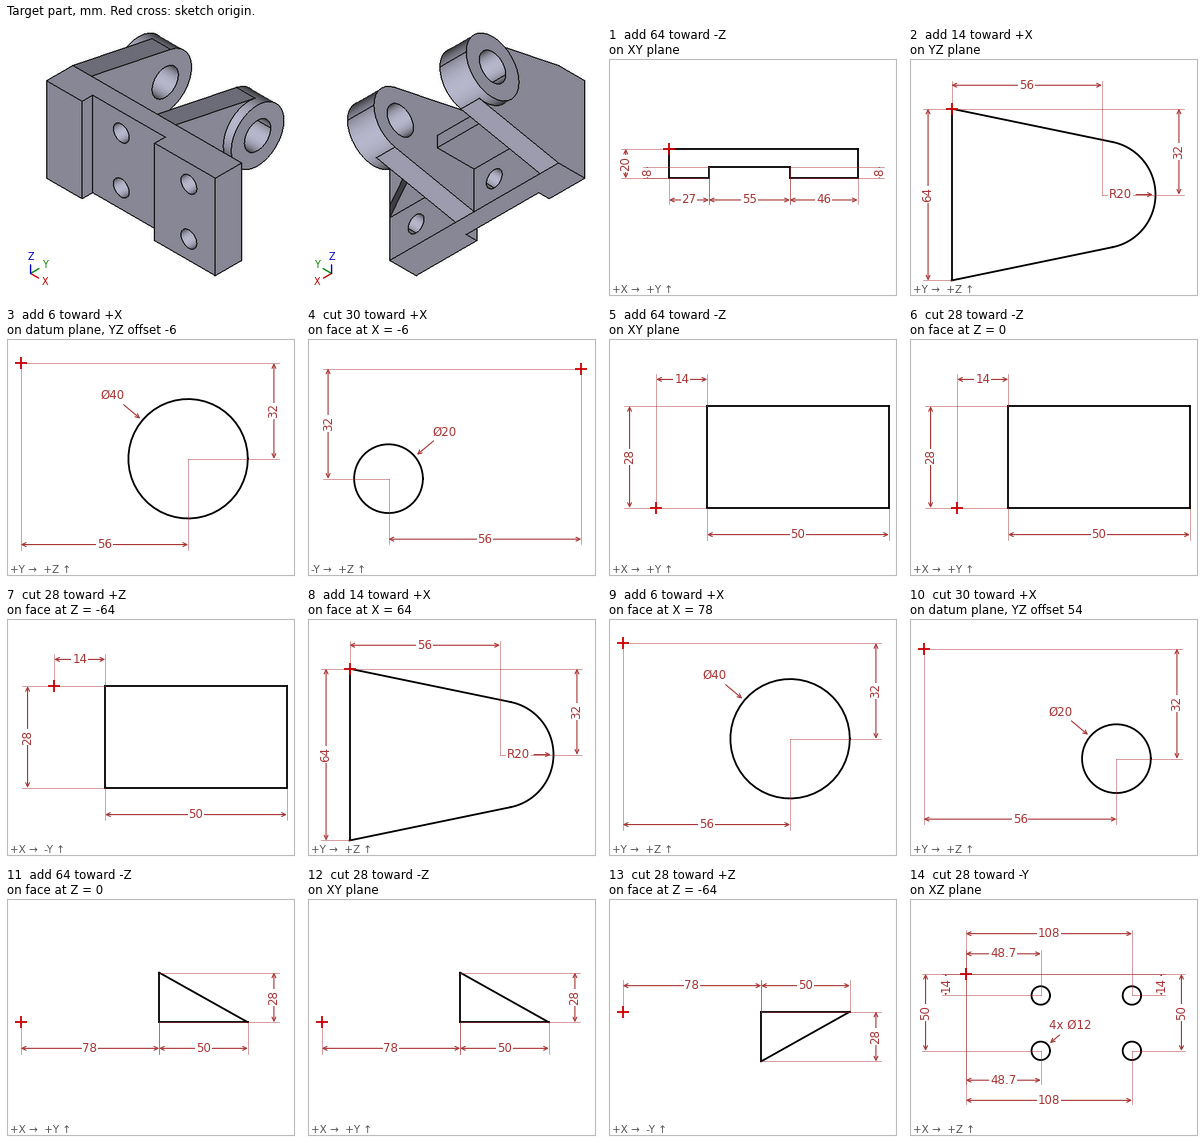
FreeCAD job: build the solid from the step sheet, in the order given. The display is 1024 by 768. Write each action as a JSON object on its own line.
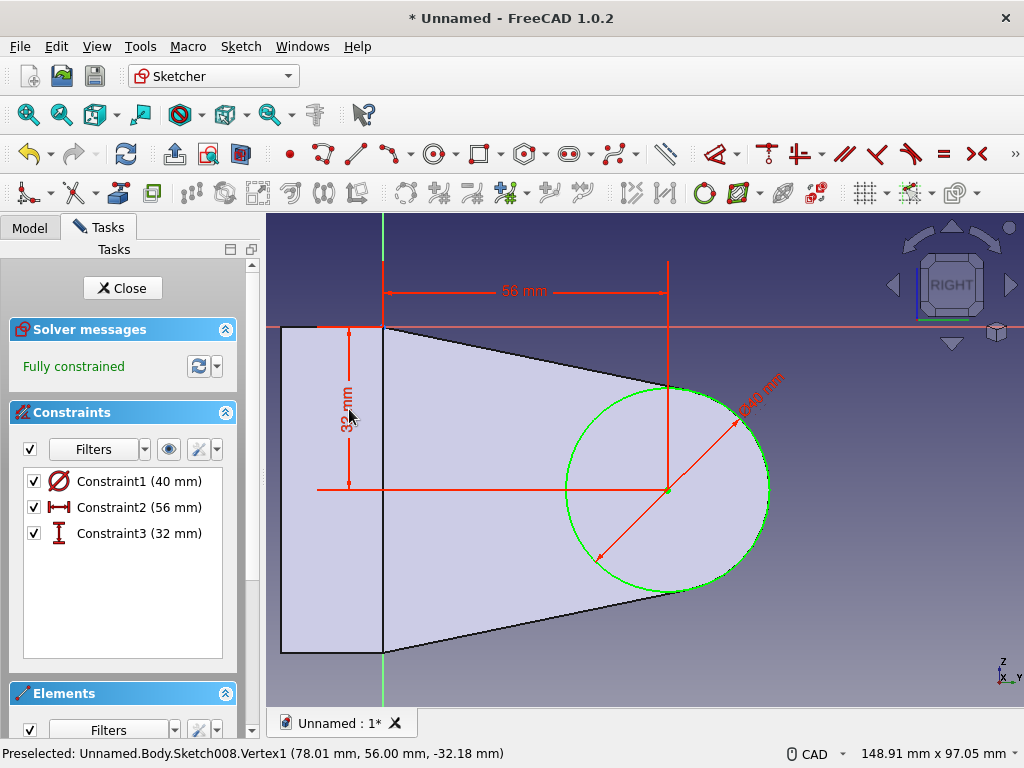
{"action": "left_click", "coordinate": [123, 288]}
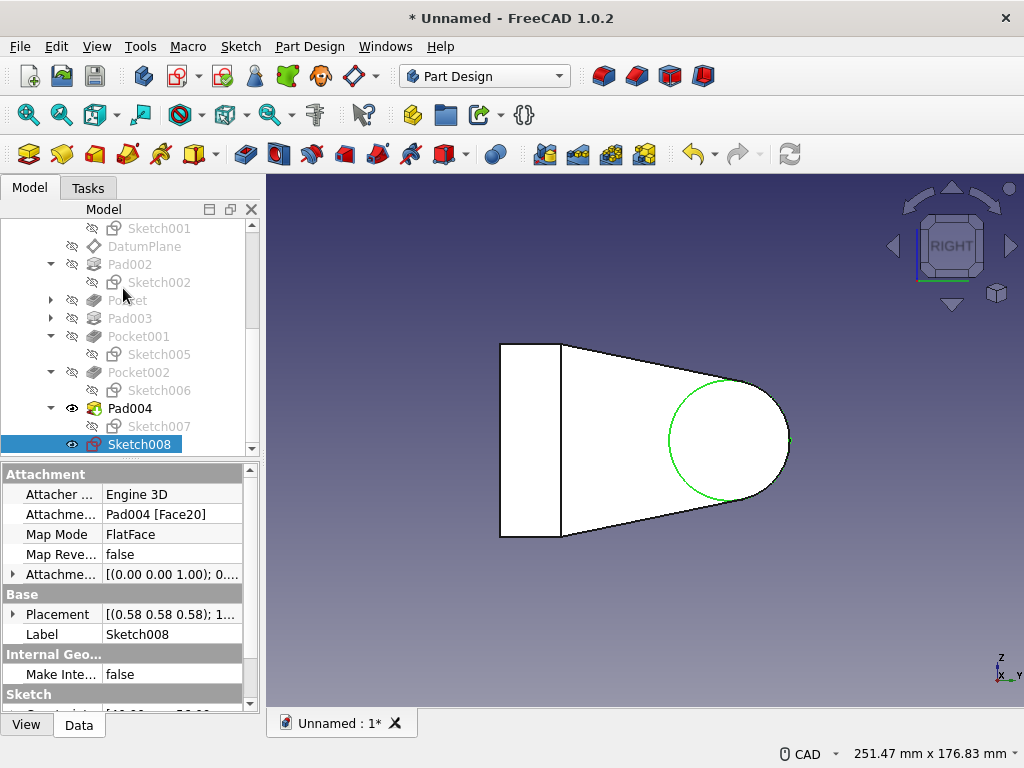
{"action": "left_click", "coordinate": [29, 154]}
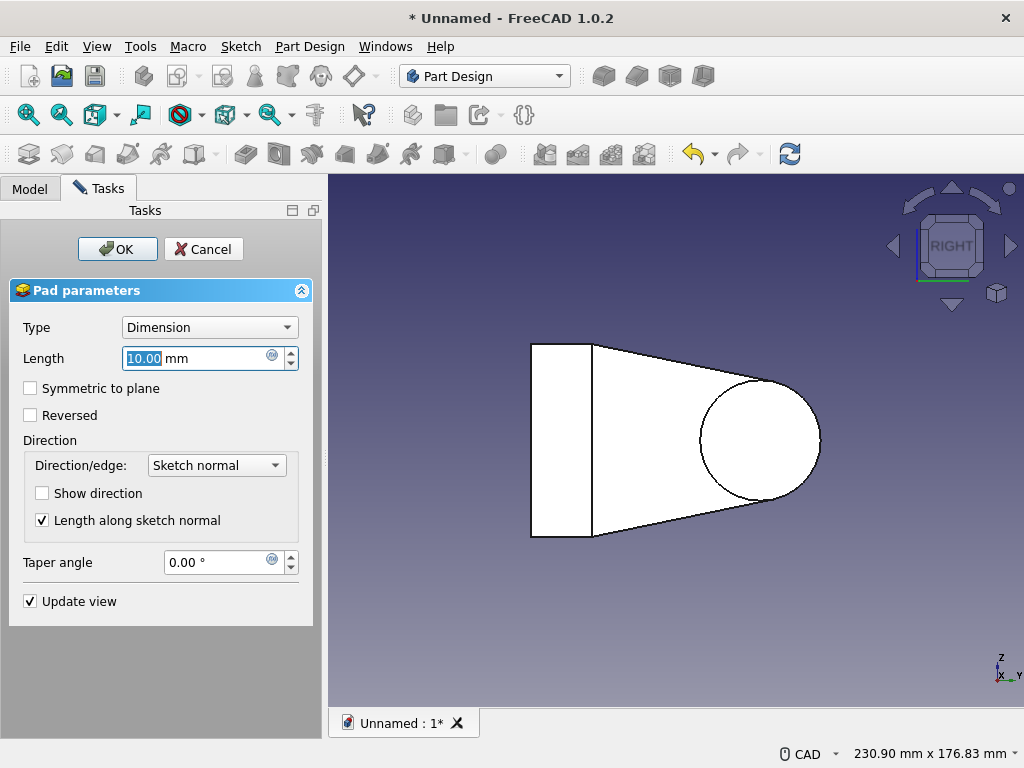
{"action": "type", "text": "6"}
{"action": "key", "text": "Tab"}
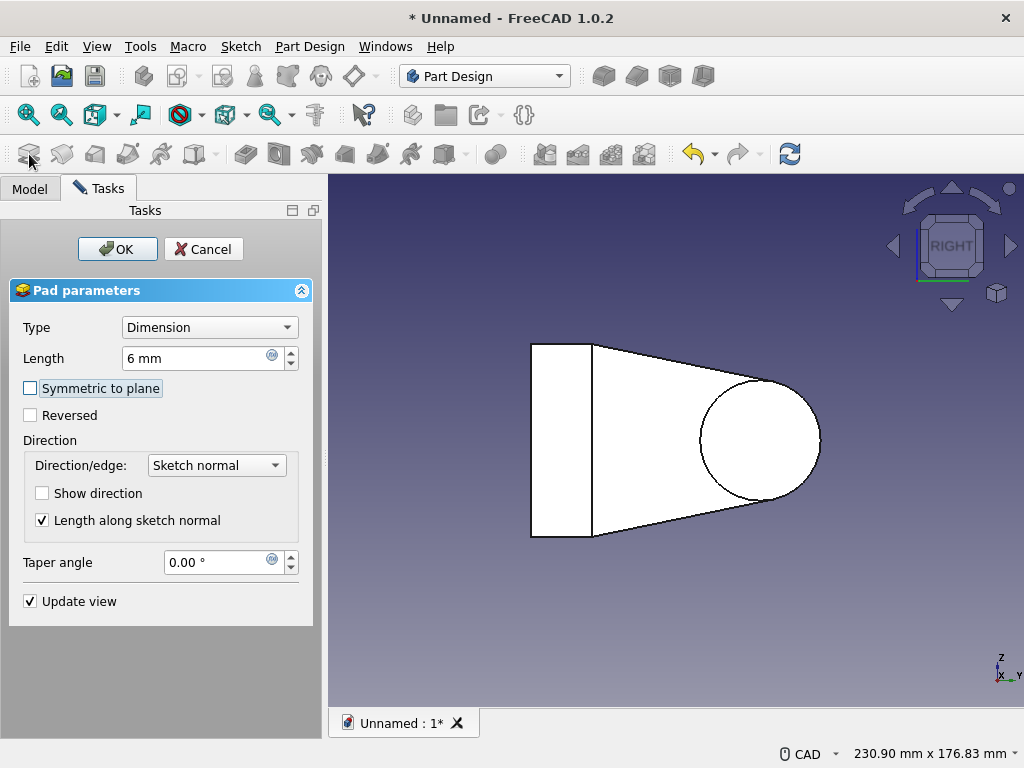
{"action": "left_click", "coordinate": [118, 249]}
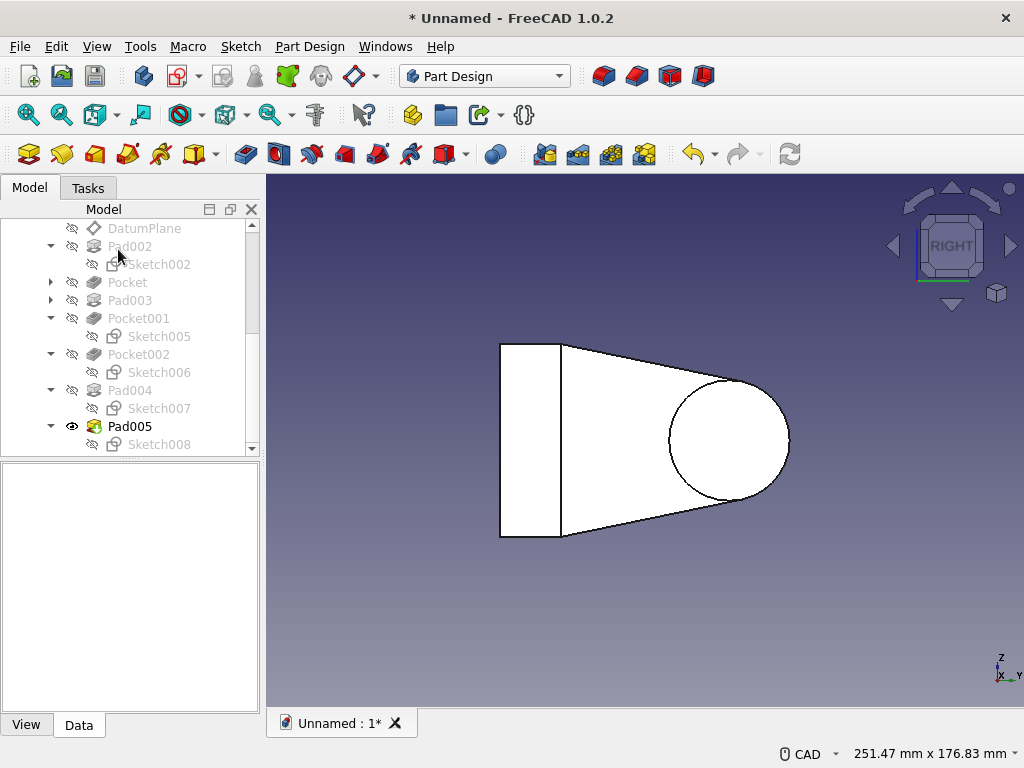
{"action": "left_click", "coordinate": [29, 116]}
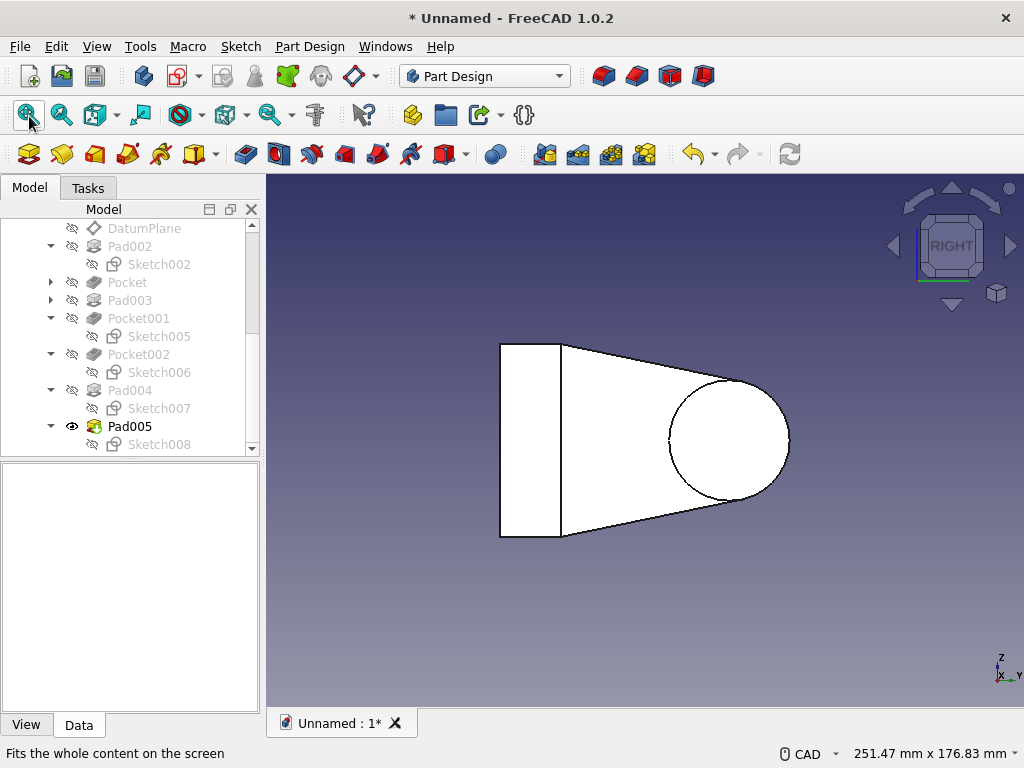
{"action": "scroll", "coordinate": [141, 332], "scroll_direction": "down", "scroll_amount": 3}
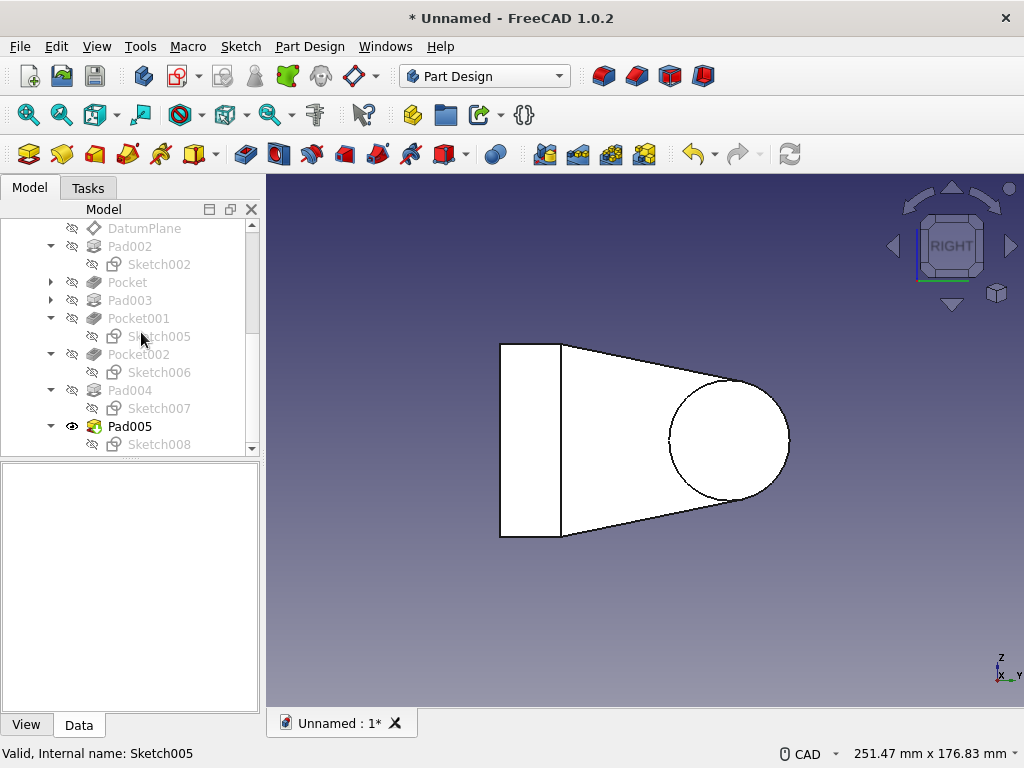
{"action": "scroll", "coordinate": [141, 332], "scroll_direction": "up", "scroll_amount": 15}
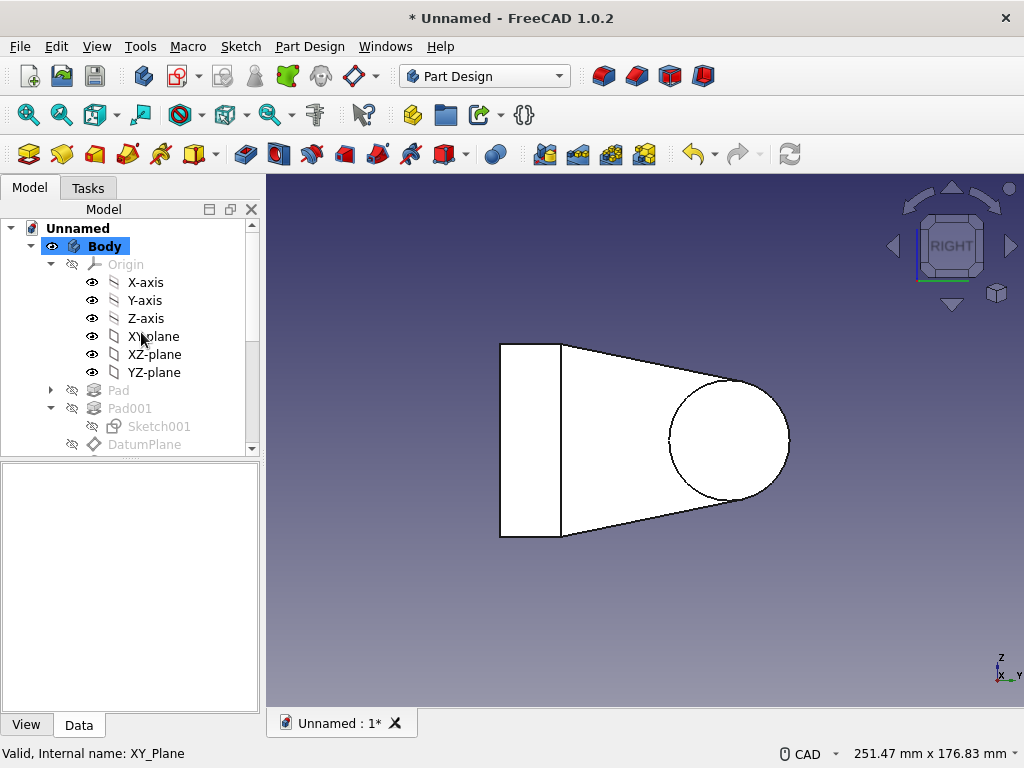
{"action": "left_click", "coordinate": [137, 372]}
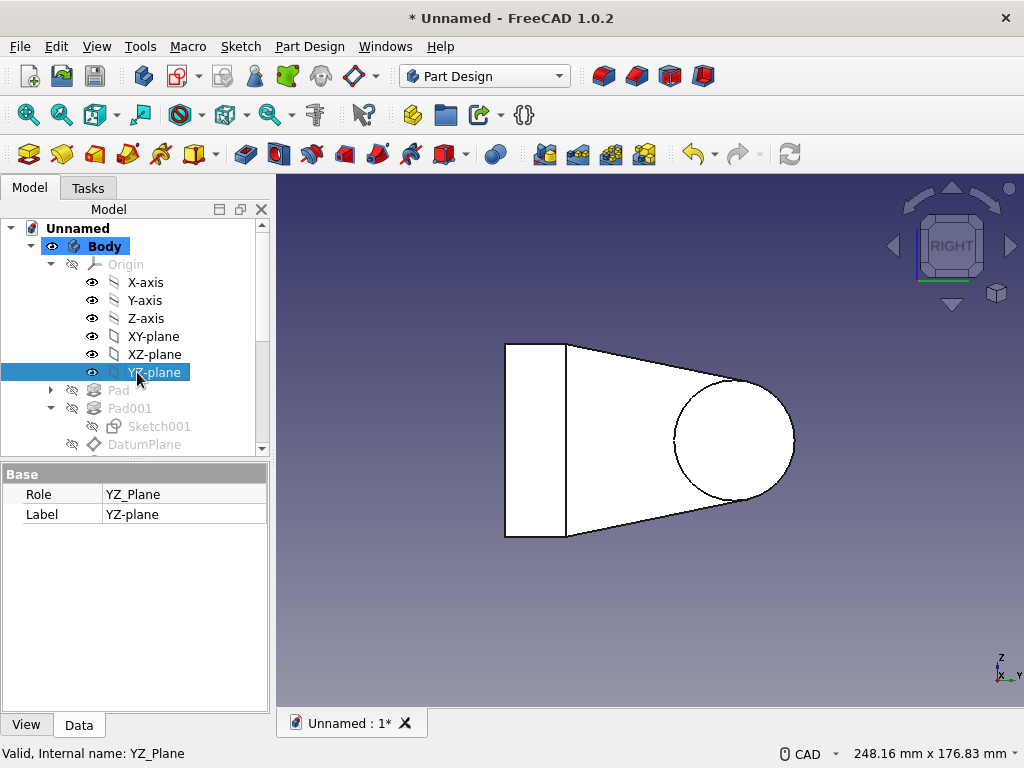
{"action": "left_click", "coordinate": [354, 76]}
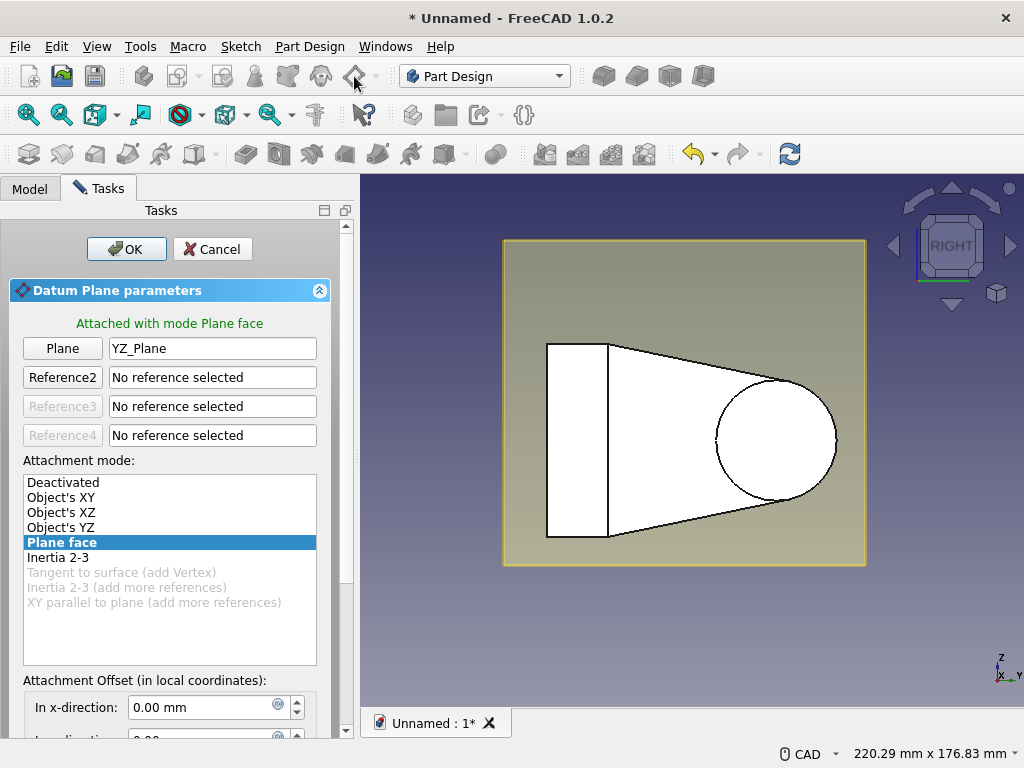
{"action": "scroll", "coordinate": [346, 479], "scroll_direction": "down", "scroll_amount": 2}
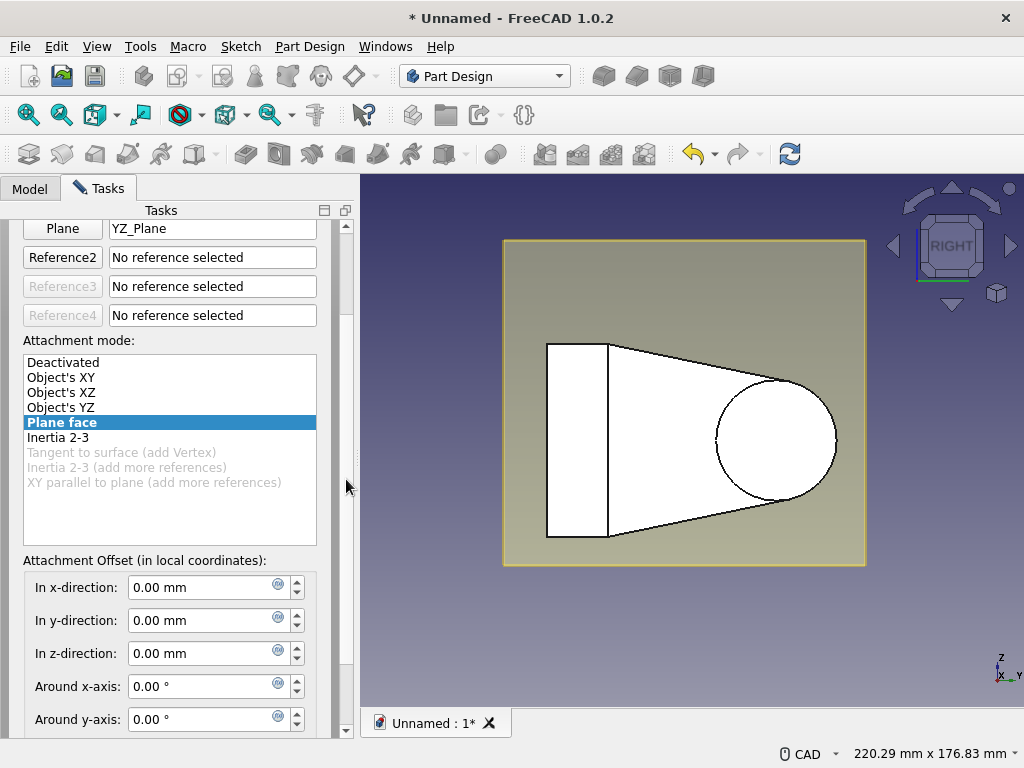
{"action": "triple_click", "coordinate": [210, 654]}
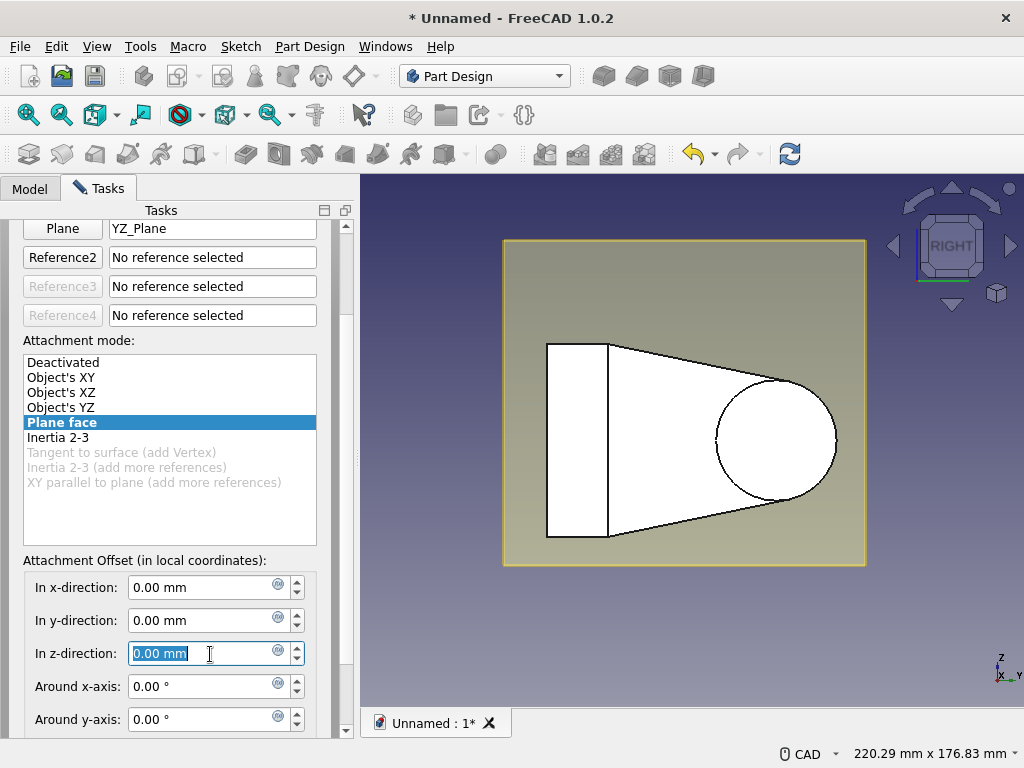
{"action": "type", "text": "54"}
{"action": "key", "text": "Tab"}